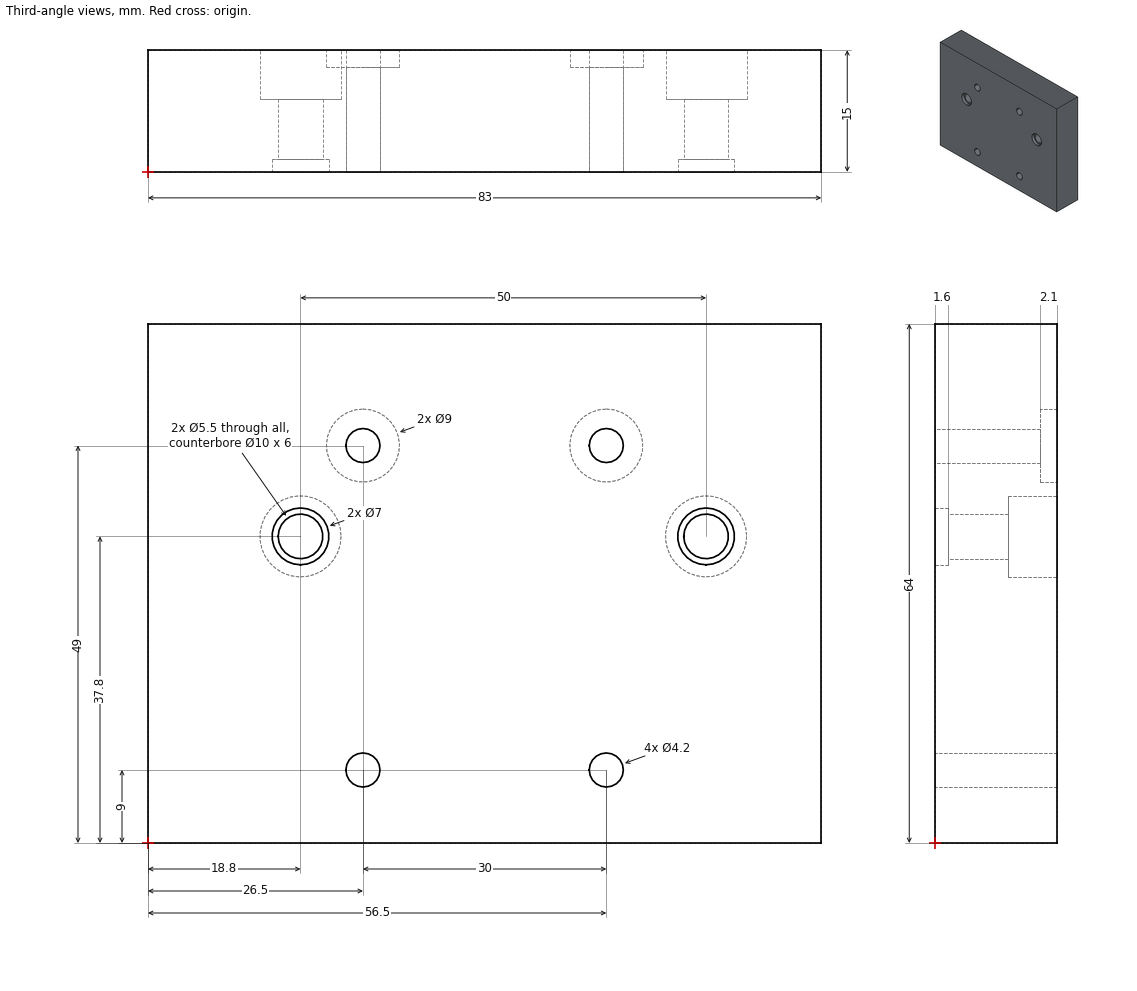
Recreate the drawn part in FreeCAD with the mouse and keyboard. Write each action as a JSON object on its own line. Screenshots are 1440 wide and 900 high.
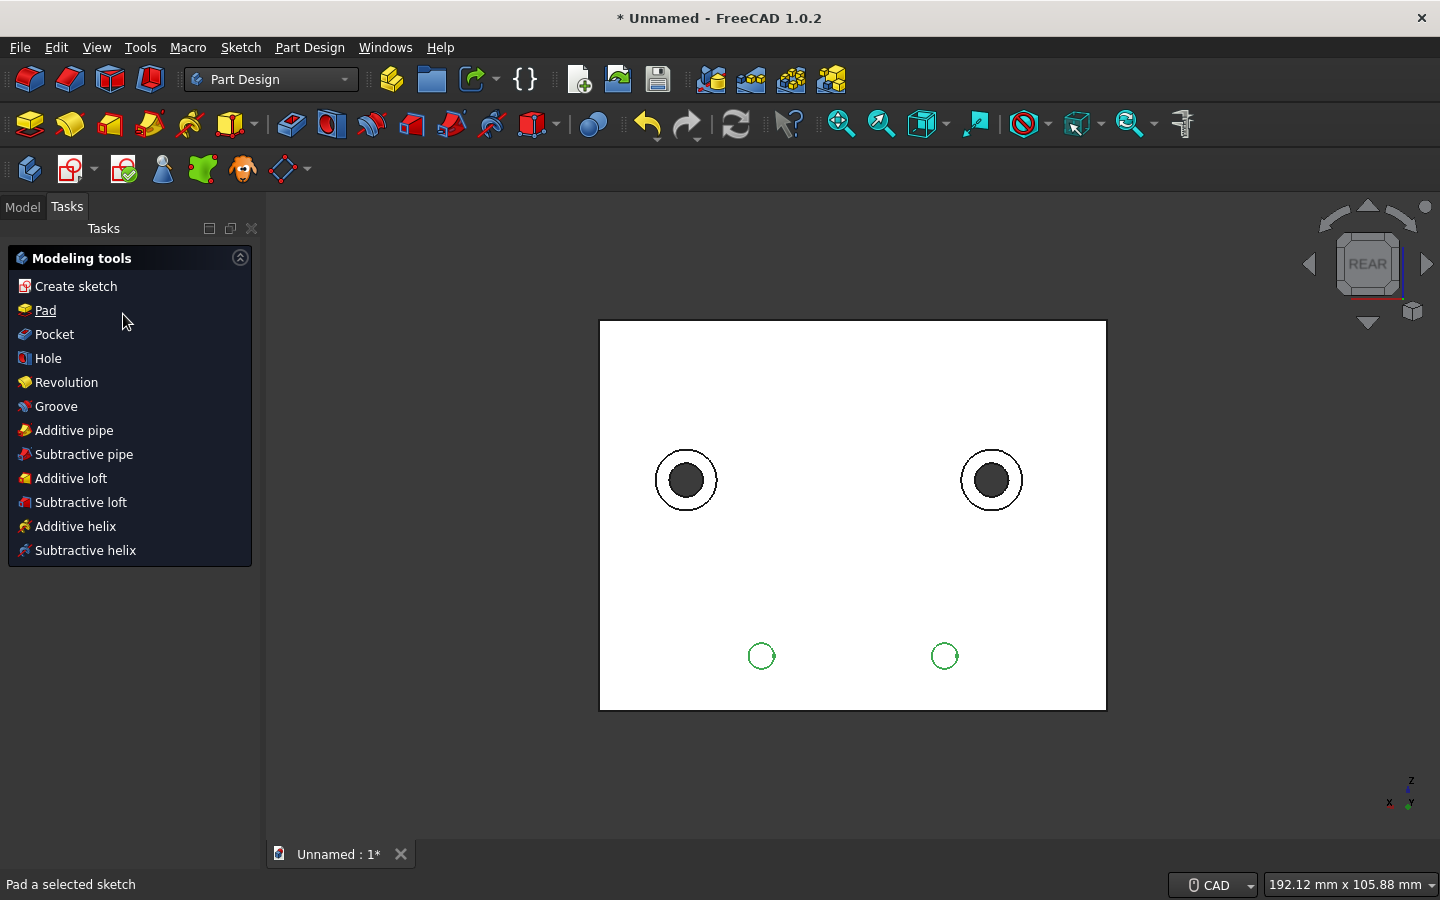
{"action": "left_click", "coordinate": [292, 124]}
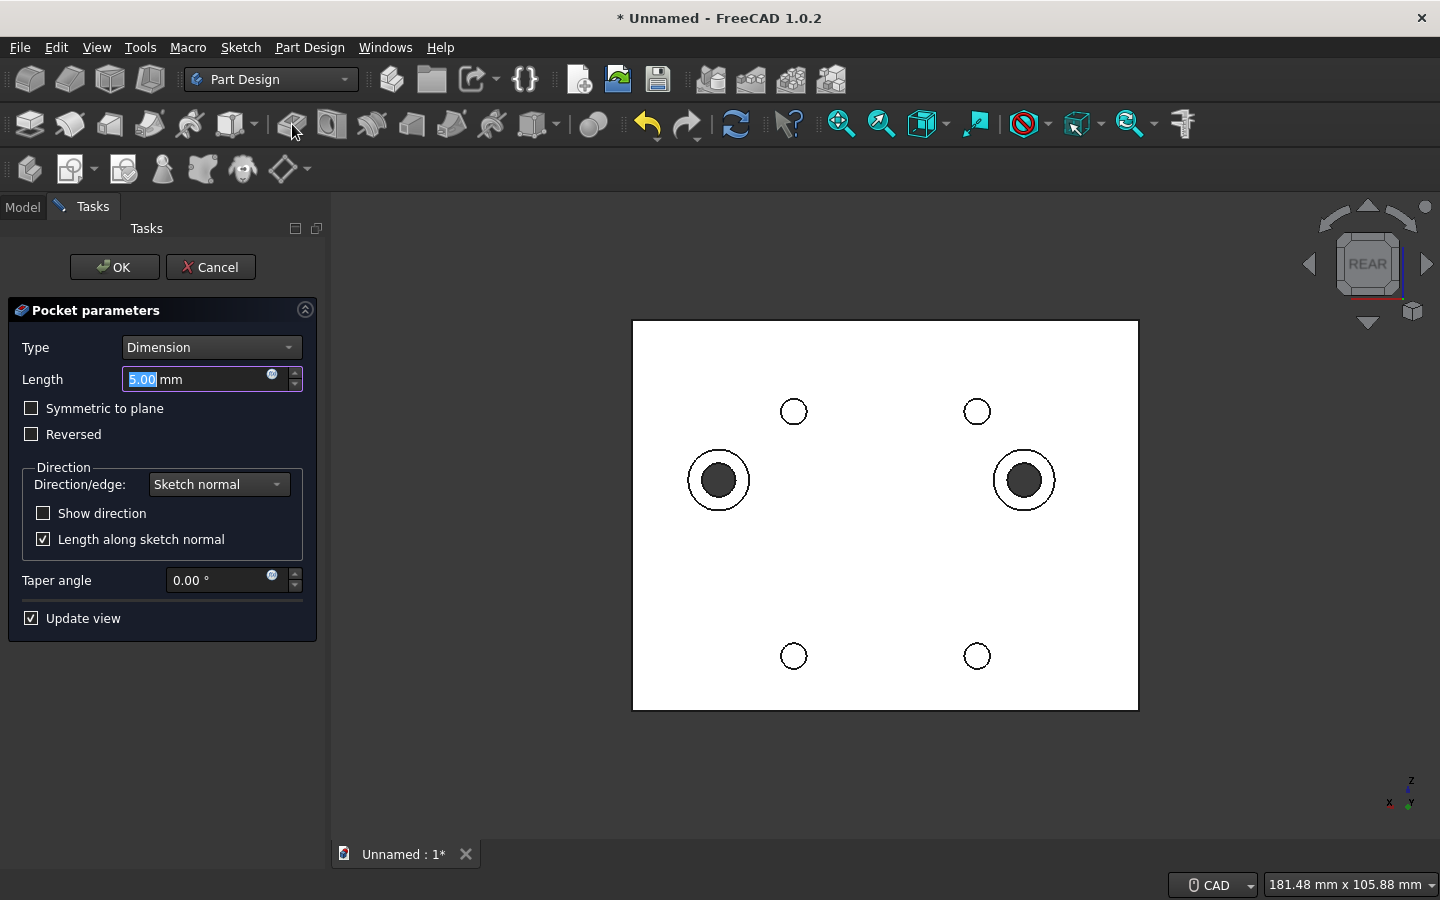
{"action": "left_click", "coordinate": [212, 348]}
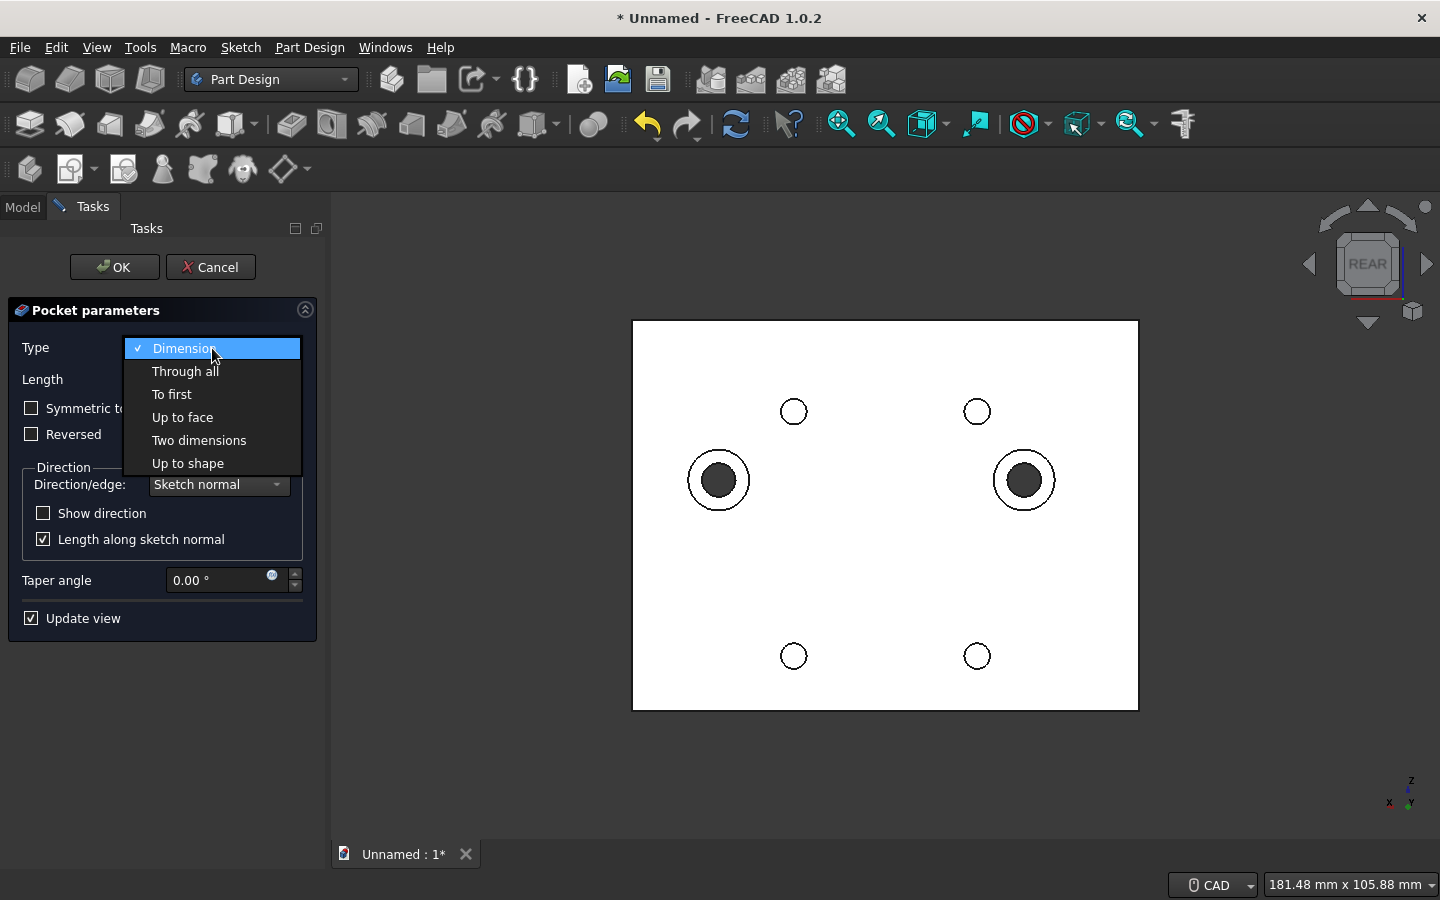
{"action": "left_click", "coordinate": [212, 372]}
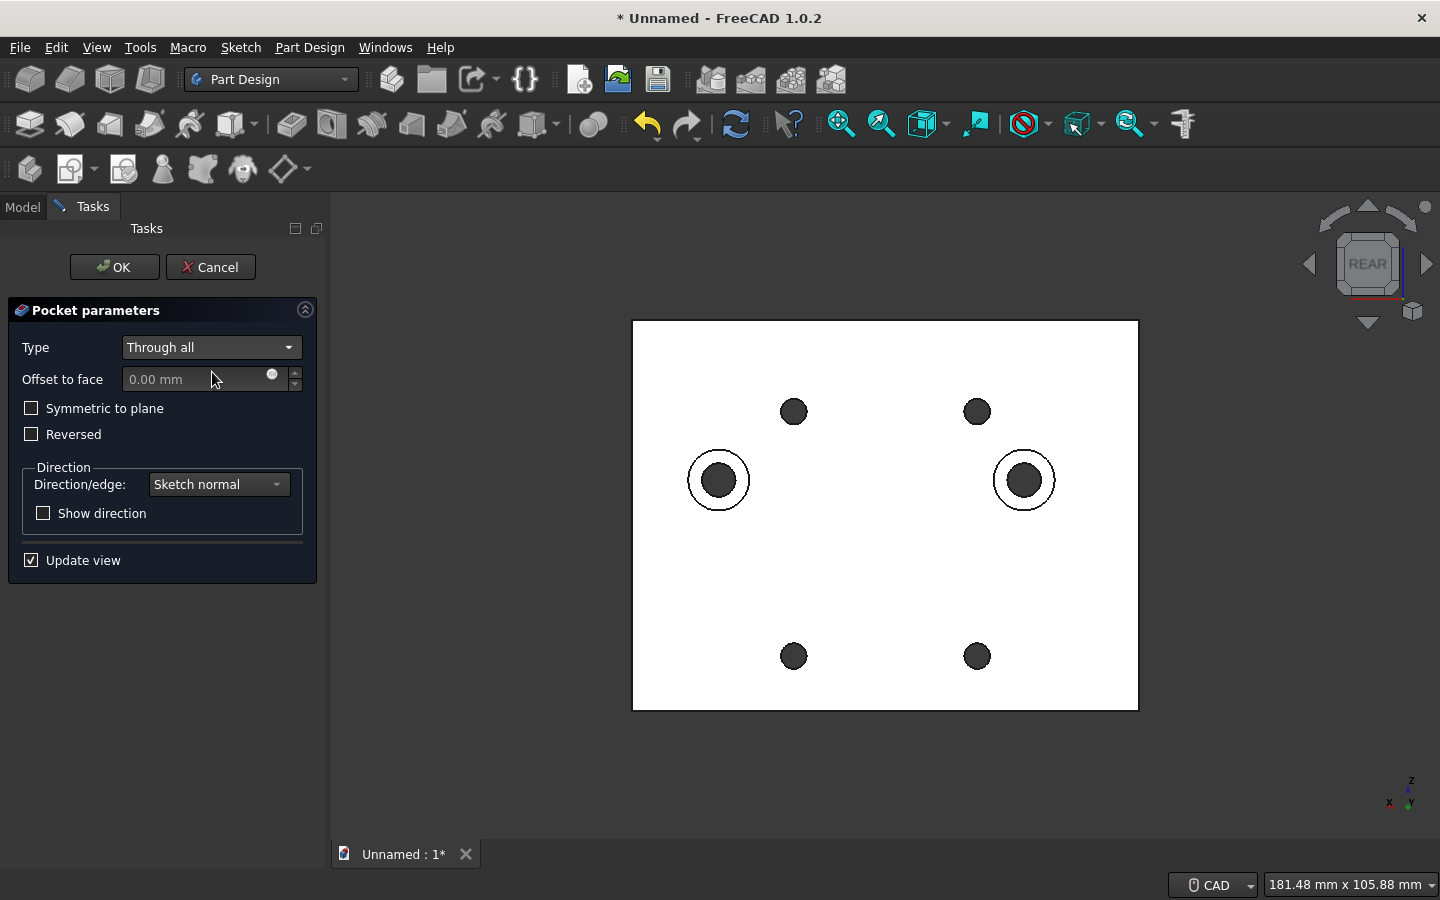
{"action": "left_click", "coordinate": [115, 267]}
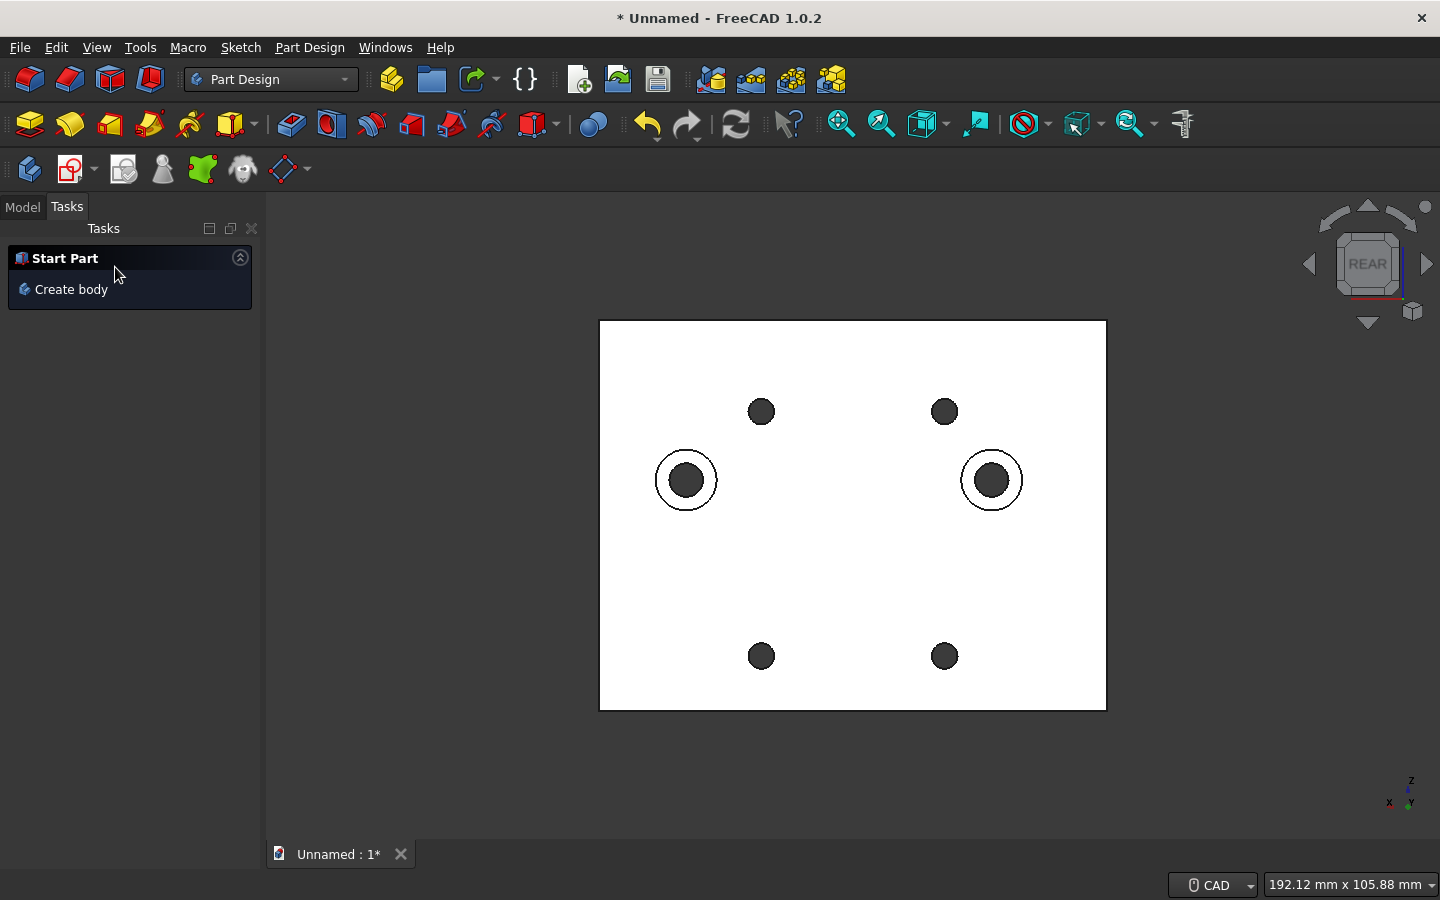
{"action": "left_click", "coordinate": [853, 515]}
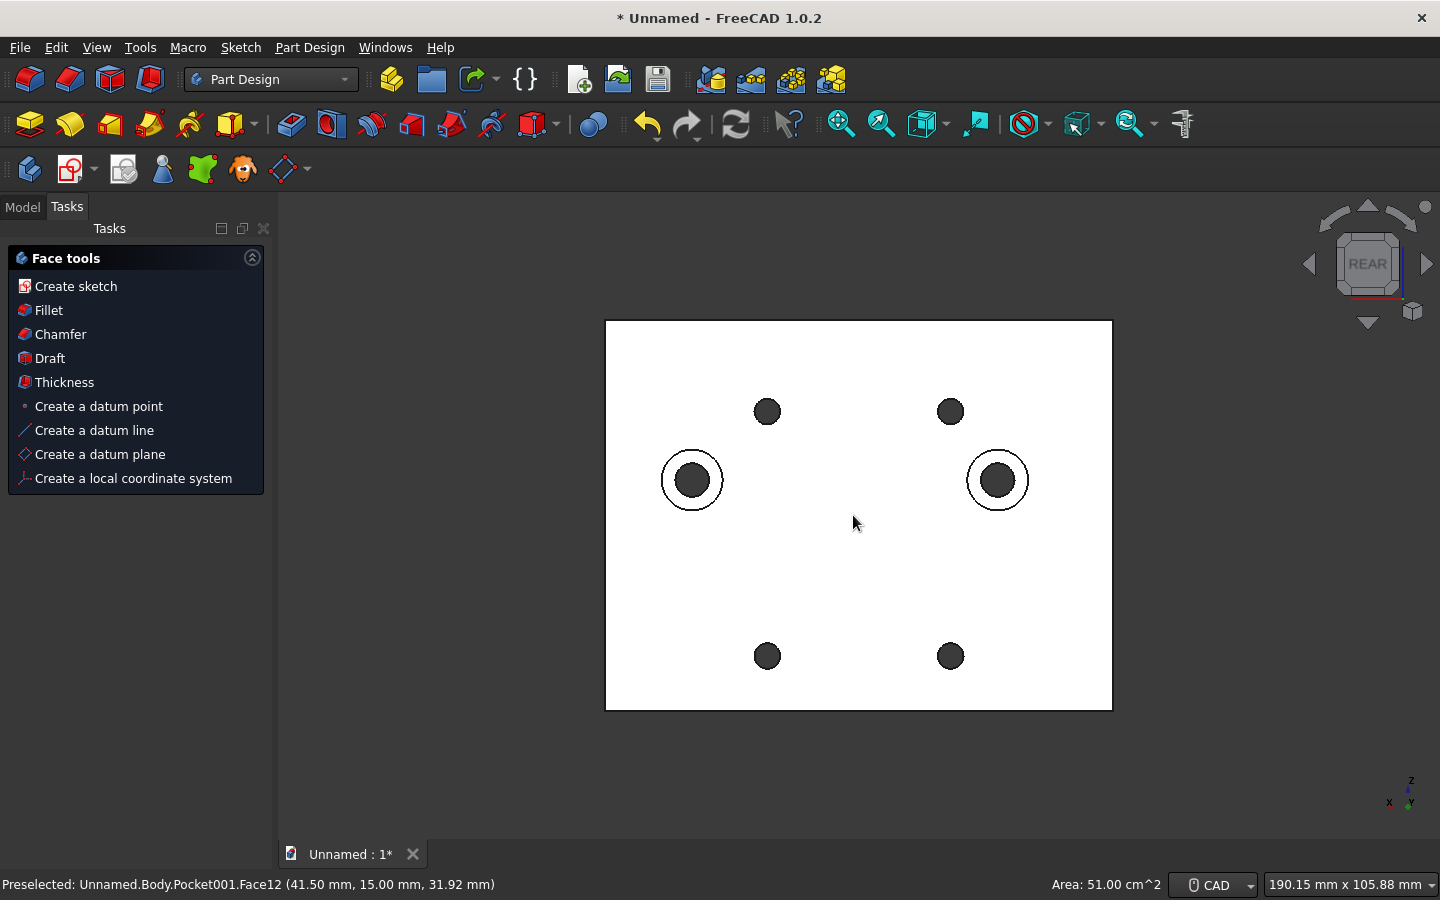
{"action": "left_click", "coordinate": [70, 170]}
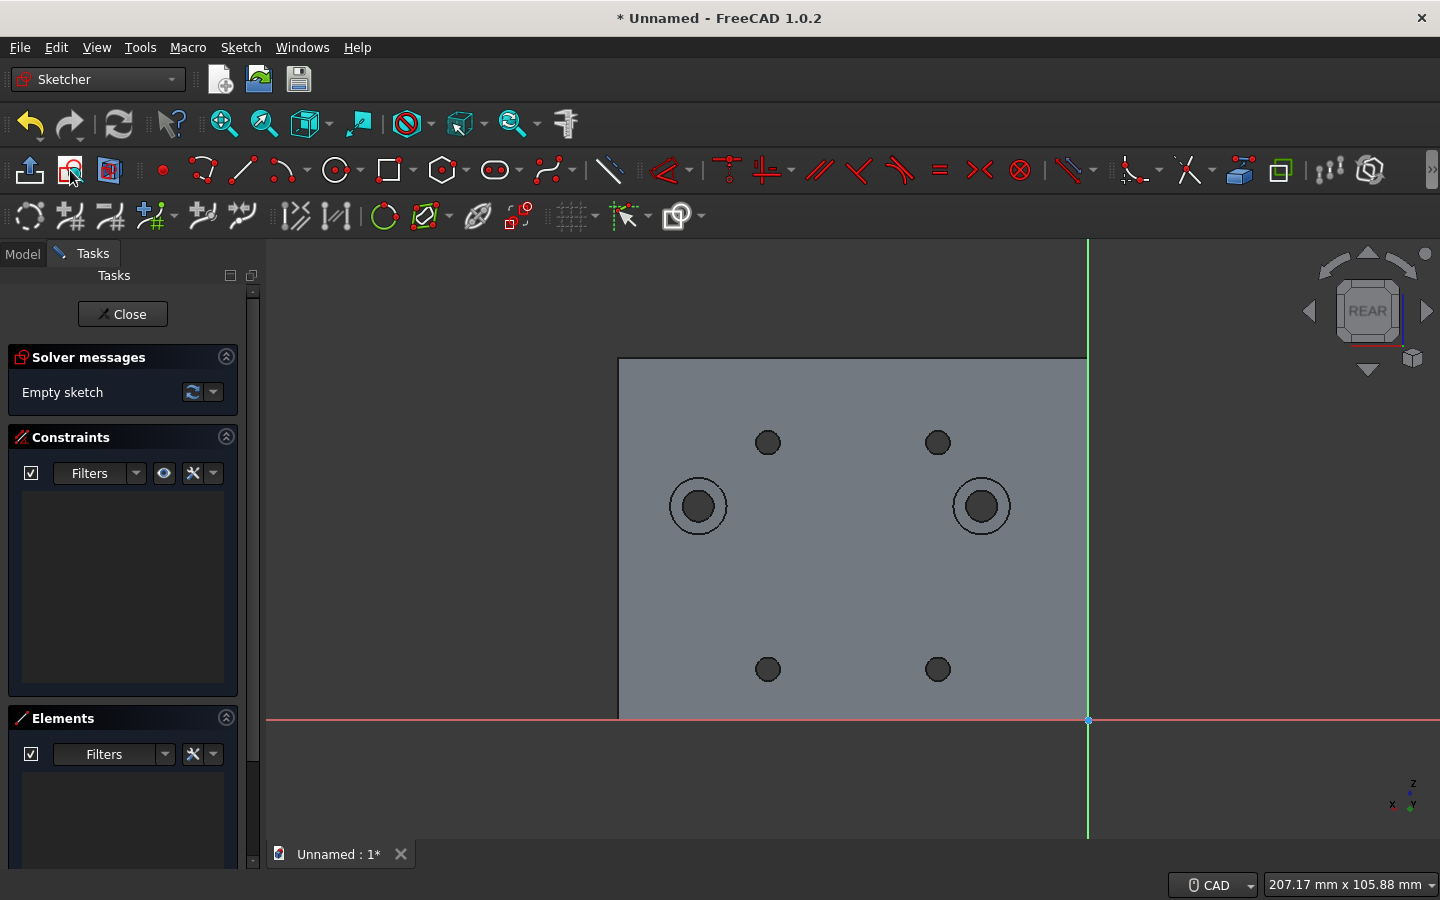
{"action": "left_click", "coordinate": [336, 170]}